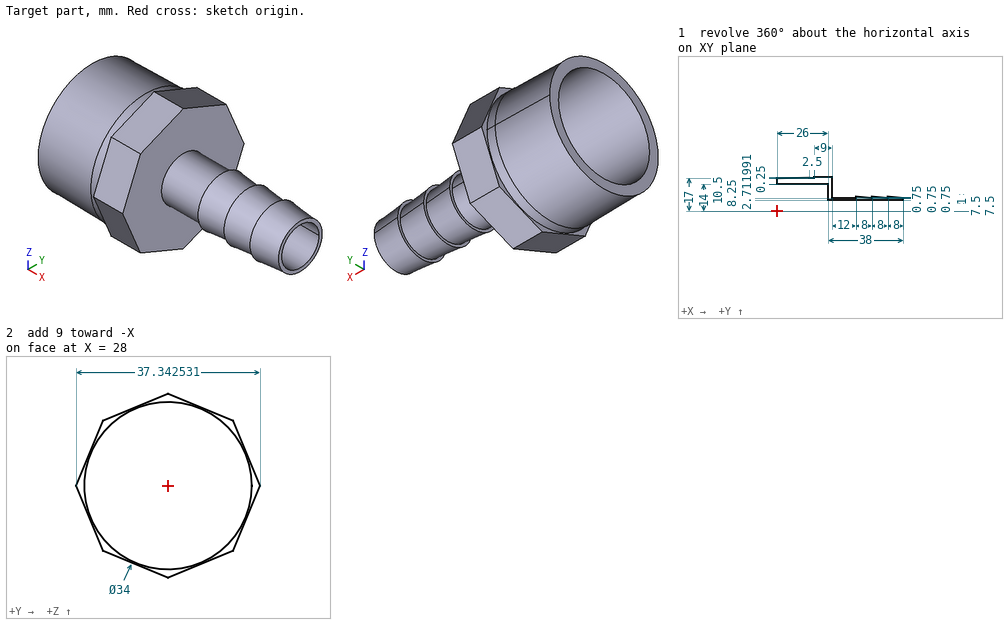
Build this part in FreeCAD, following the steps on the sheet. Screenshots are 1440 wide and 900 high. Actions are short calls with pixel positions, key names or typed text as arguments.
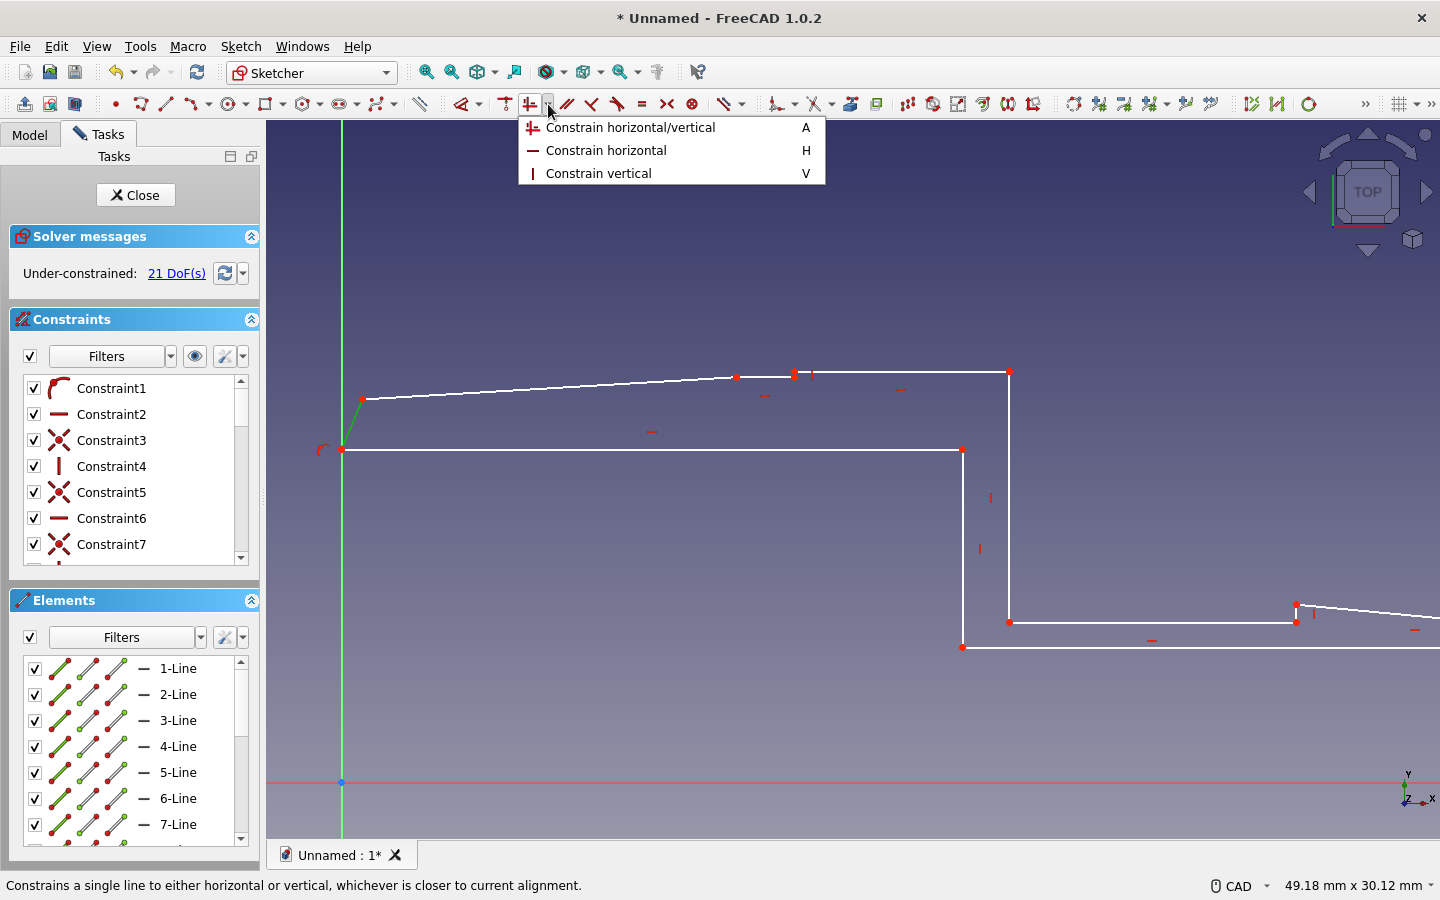
click(672, 174)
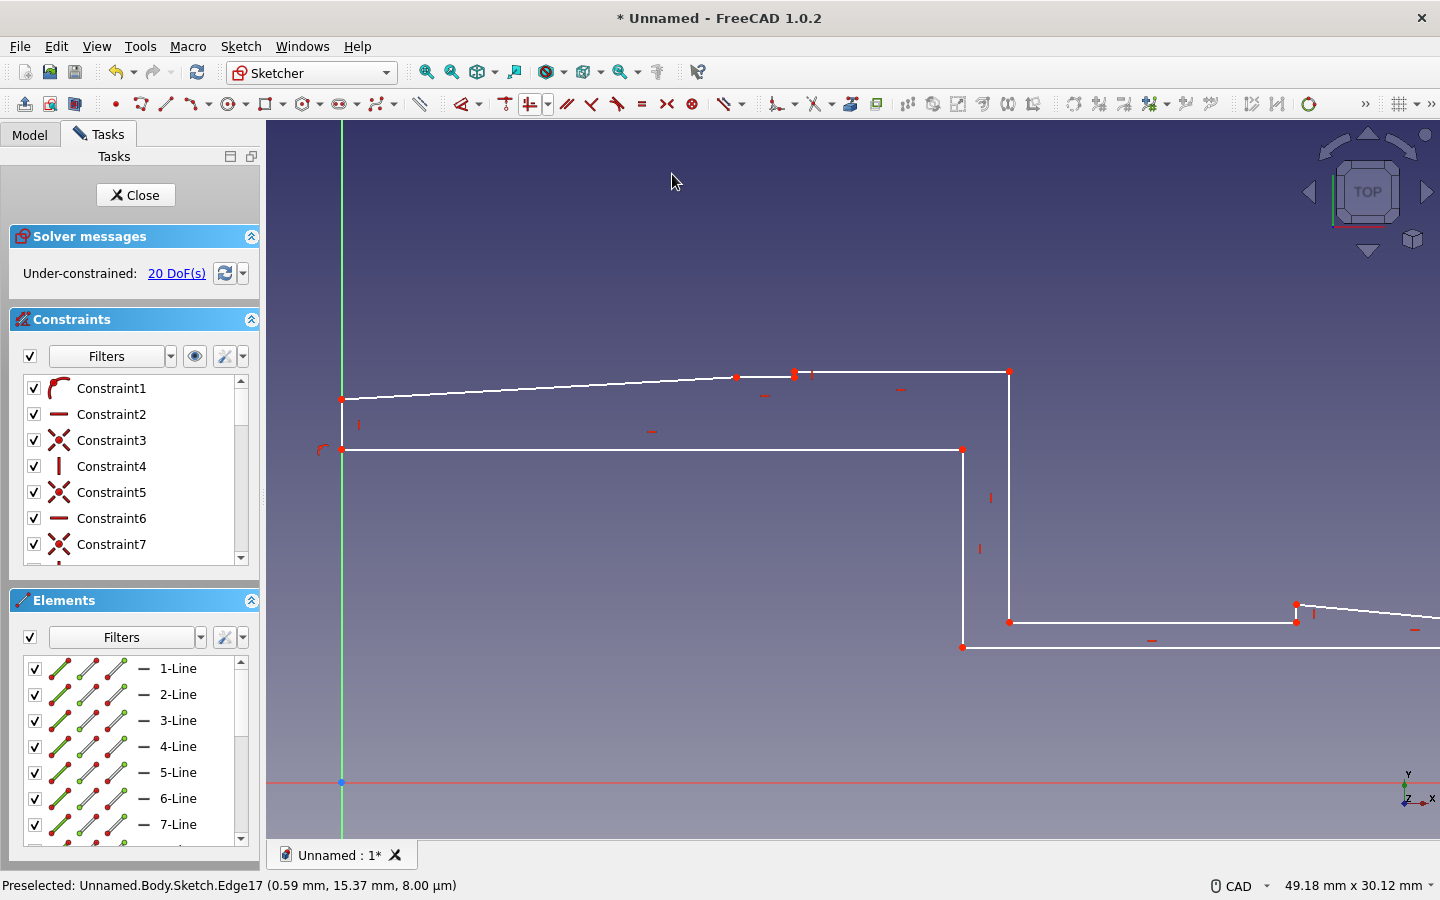
click(460, 104)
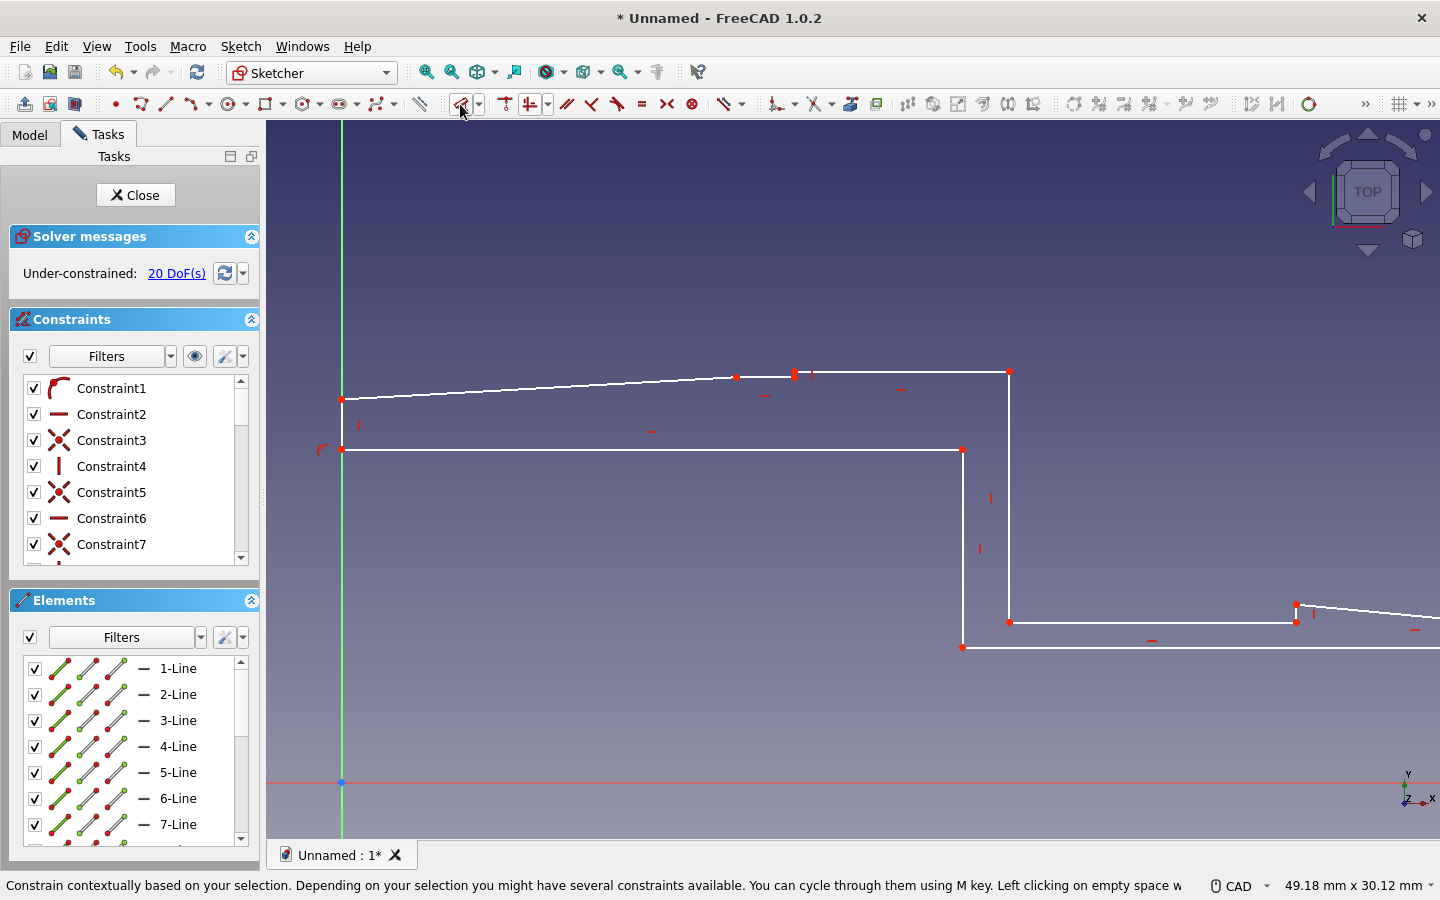
scroll(523, 400, down, 4)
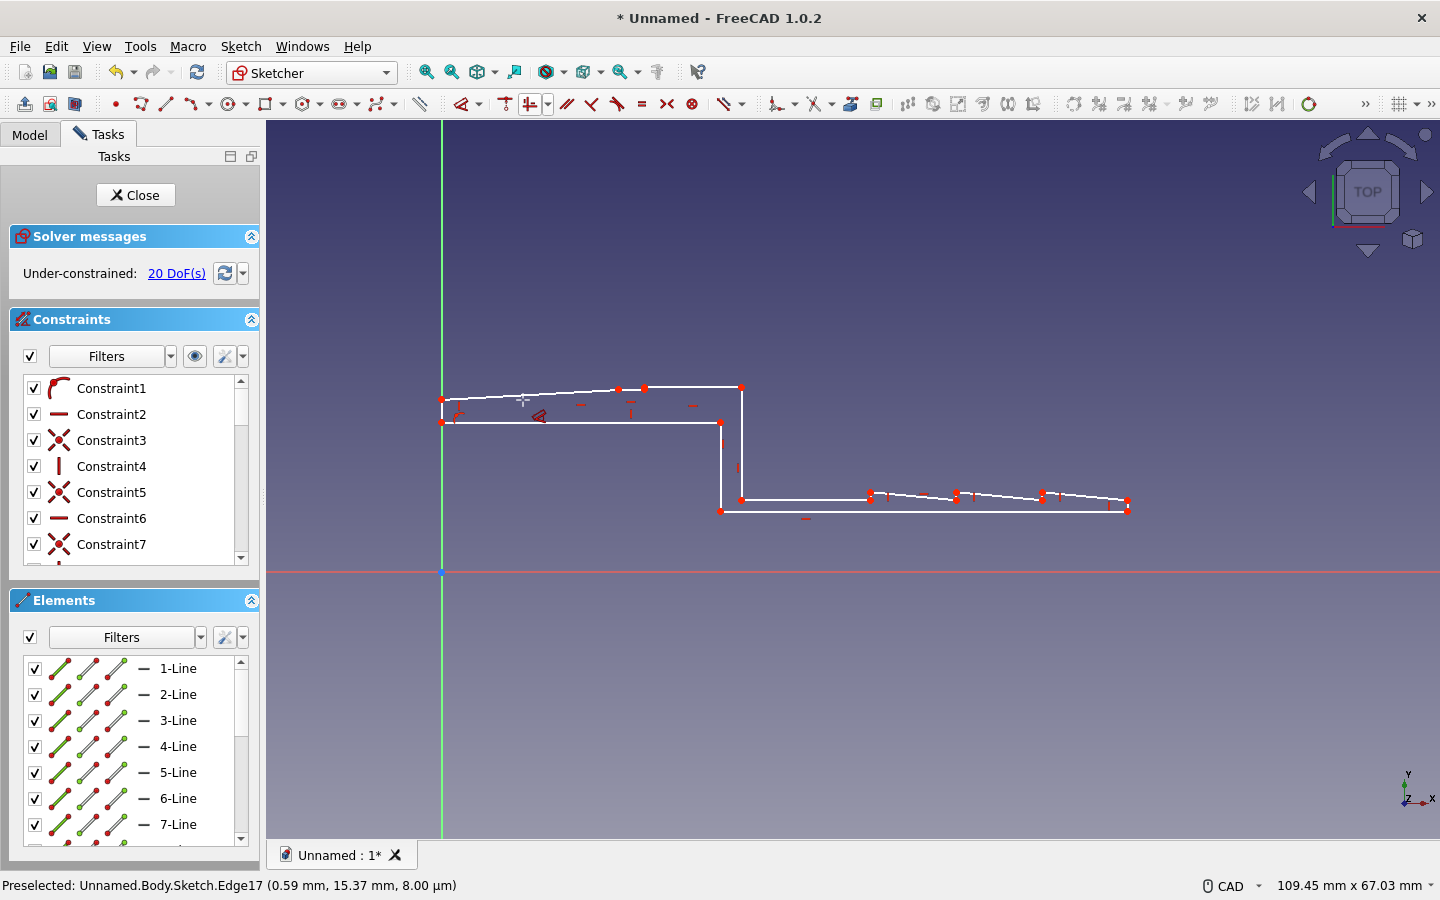
scroll(1128, 507, up, 7)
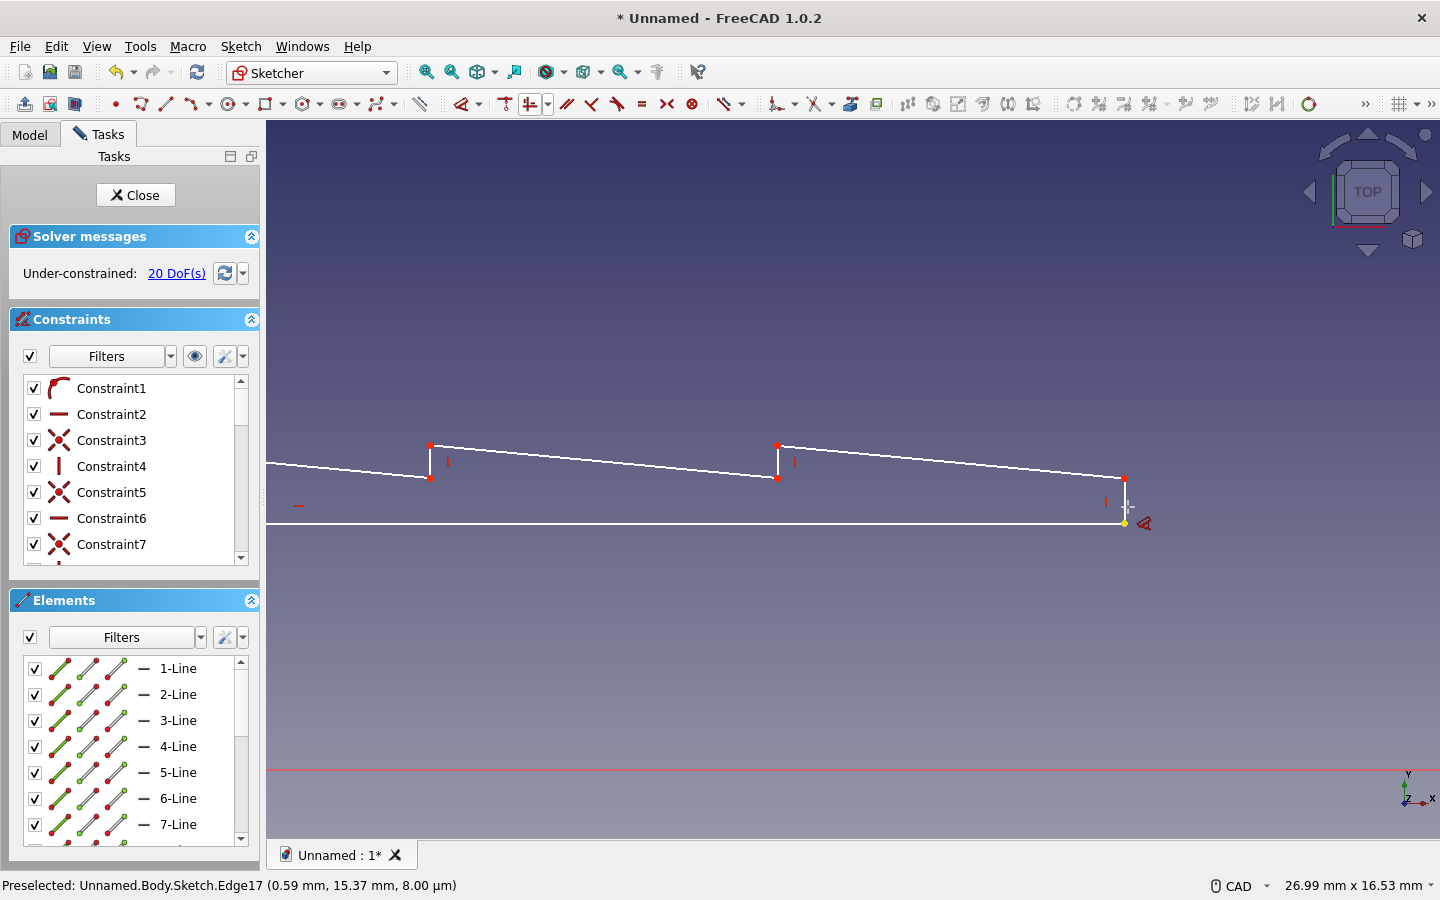
click(1125, 506)
click(1159, 501)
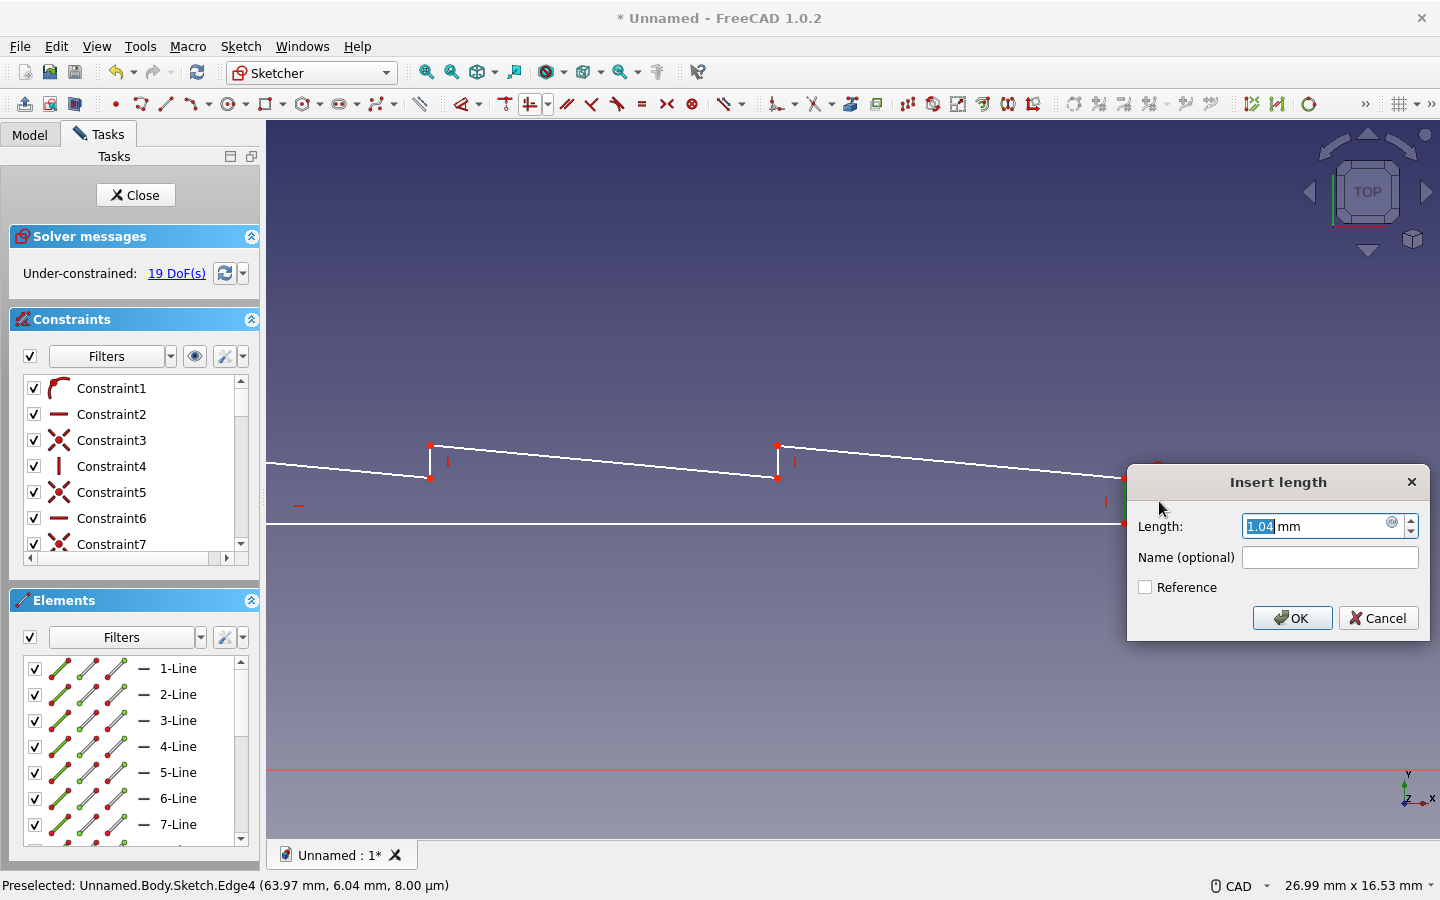
text(1)
key(Return)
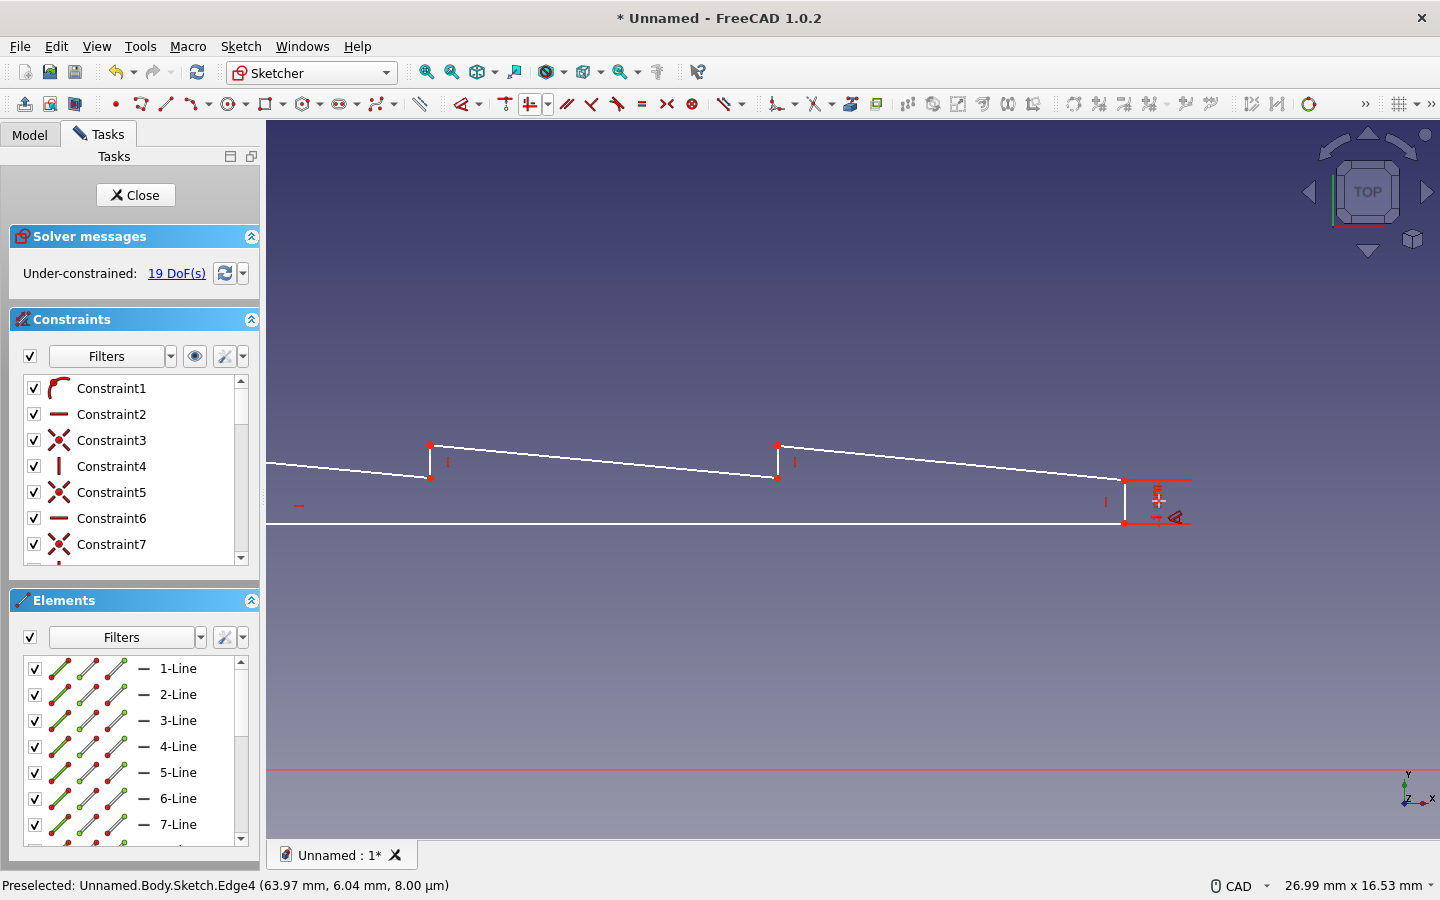
scroll(1128, 507, down, 7)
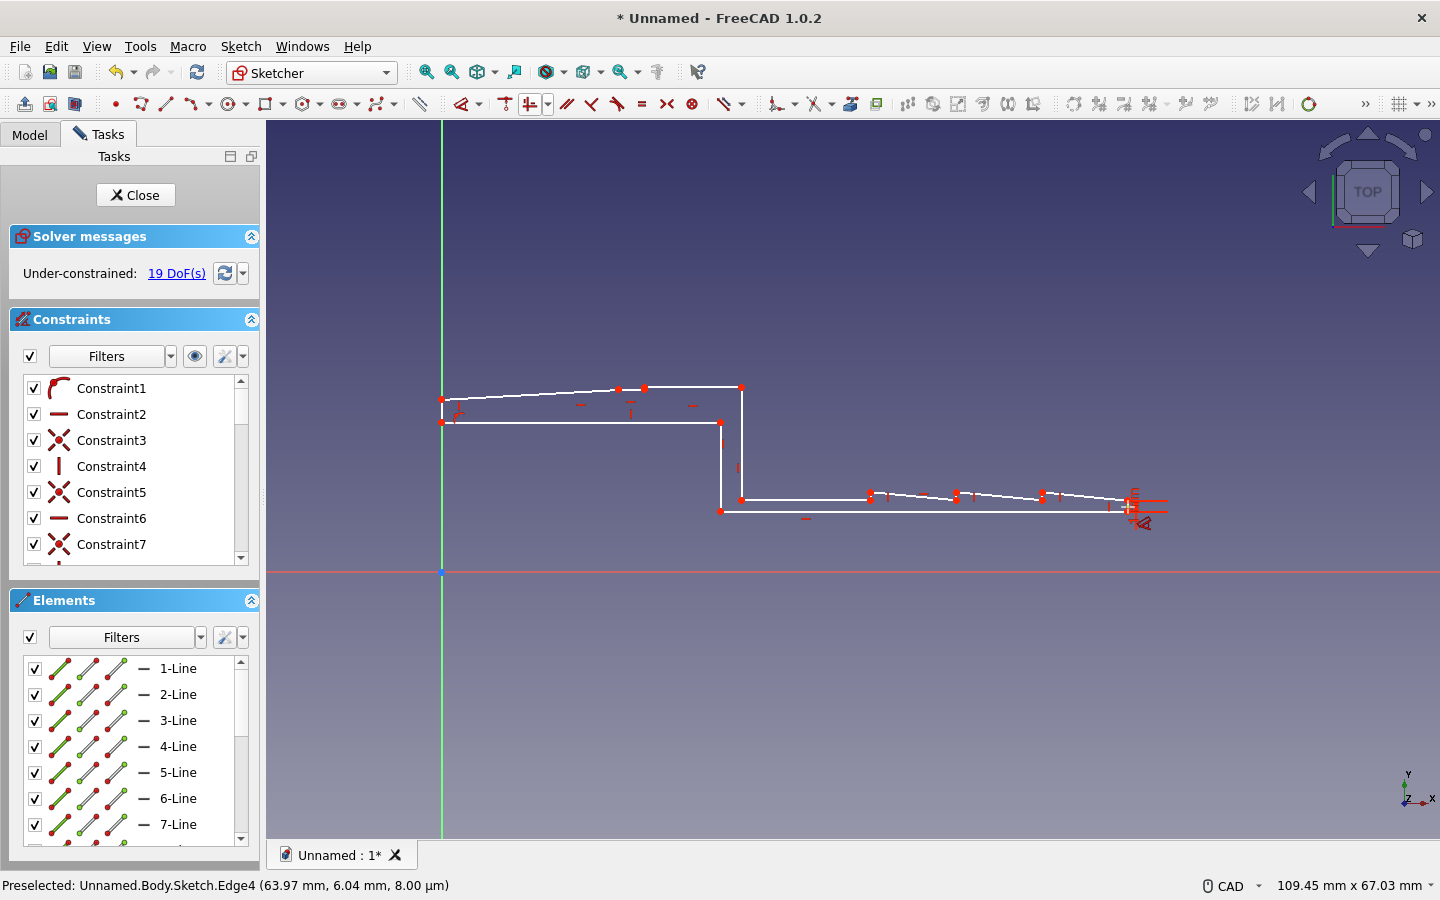
click(713, 387)
click(693, 353)